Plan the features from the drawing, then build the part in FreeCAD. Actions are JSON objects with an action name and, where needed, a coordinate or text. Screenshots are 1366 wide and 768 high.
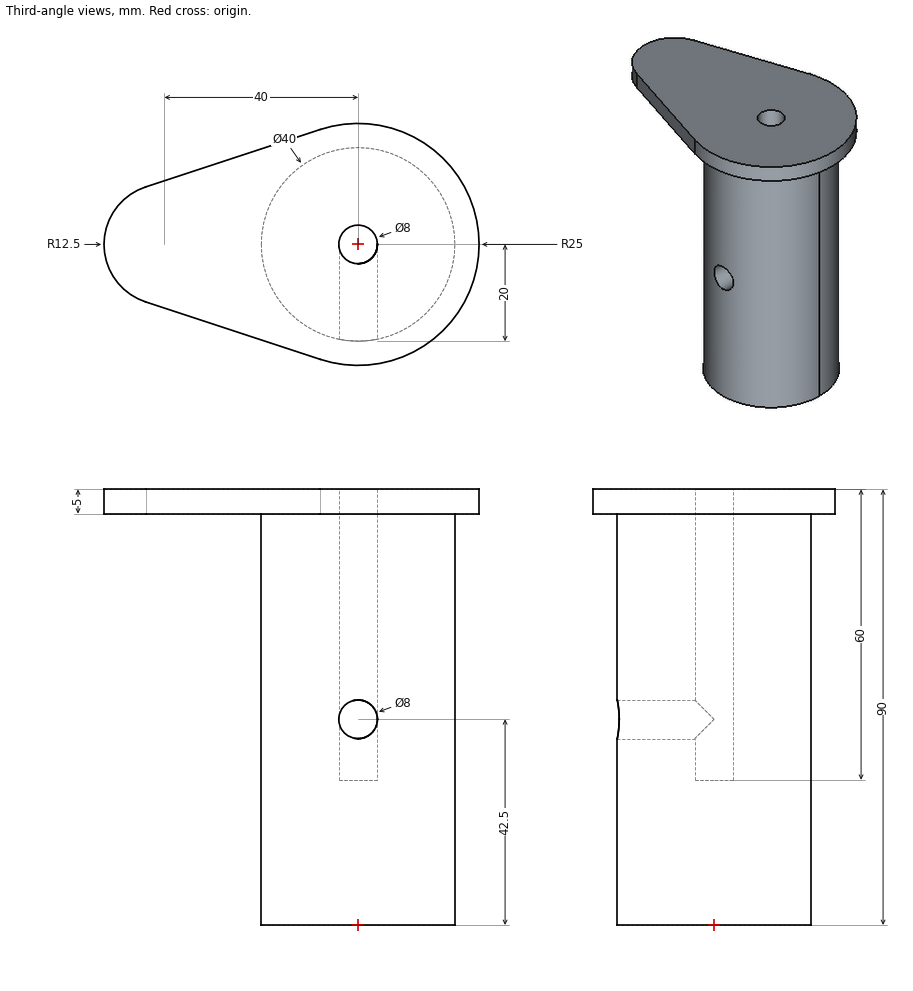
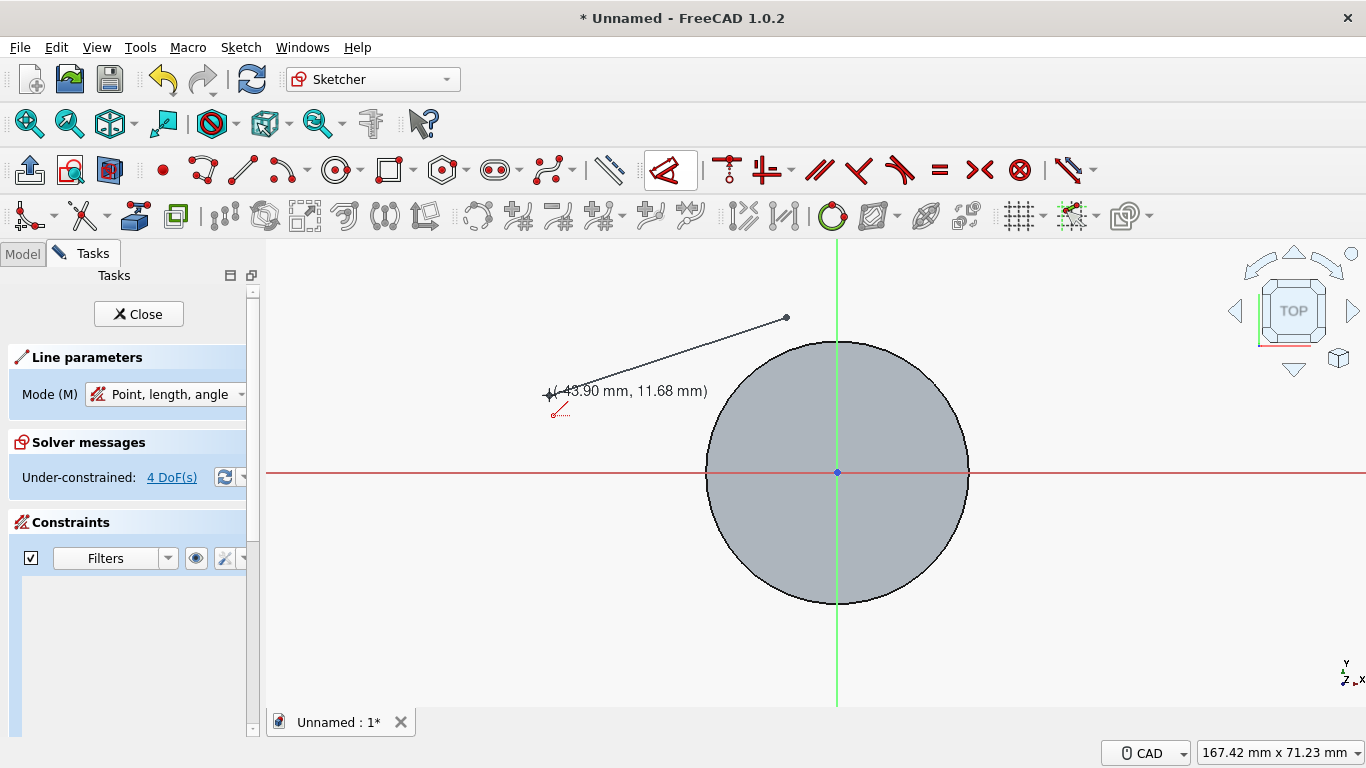
{"action": "left_click", "coordinate": [549, 551]}
{"action": "left_click", "coordinate": [786, 629]}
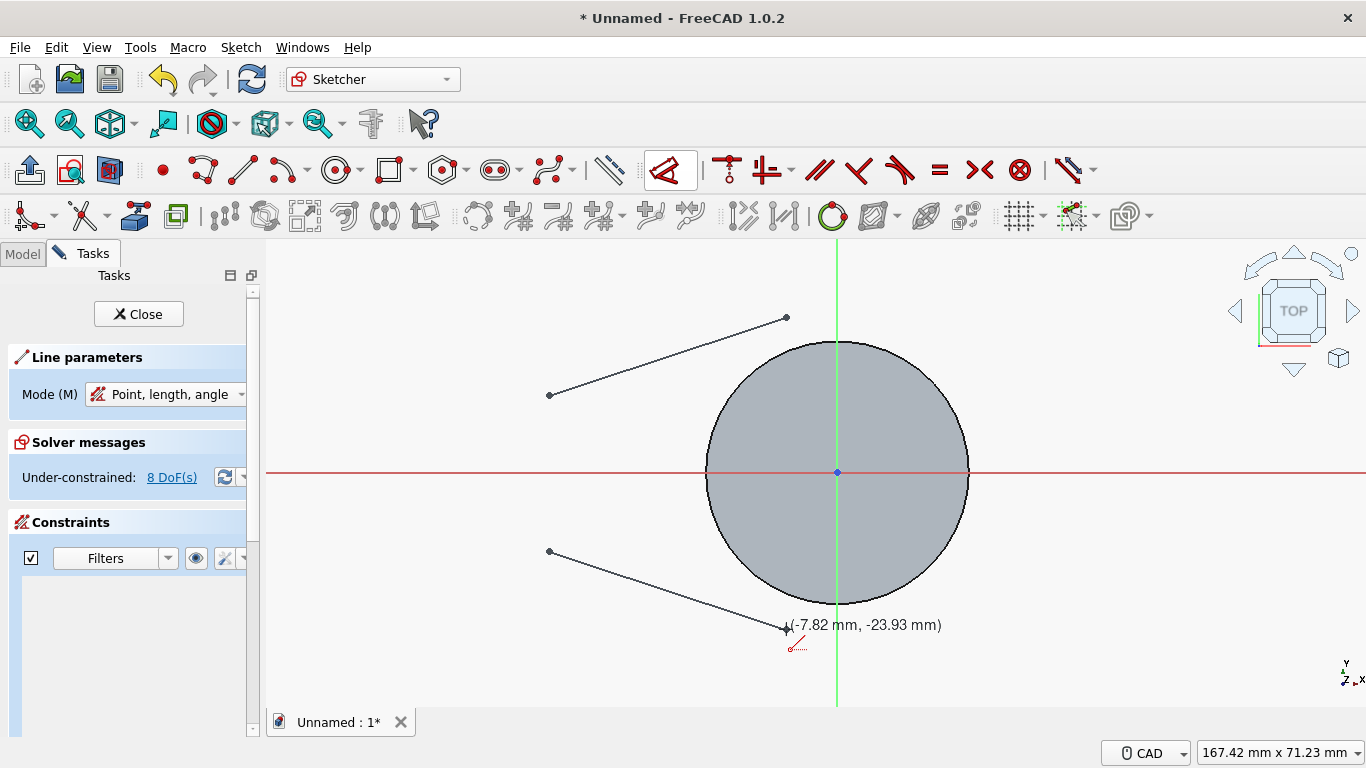
{"action": "key", "text": "g 3 a"}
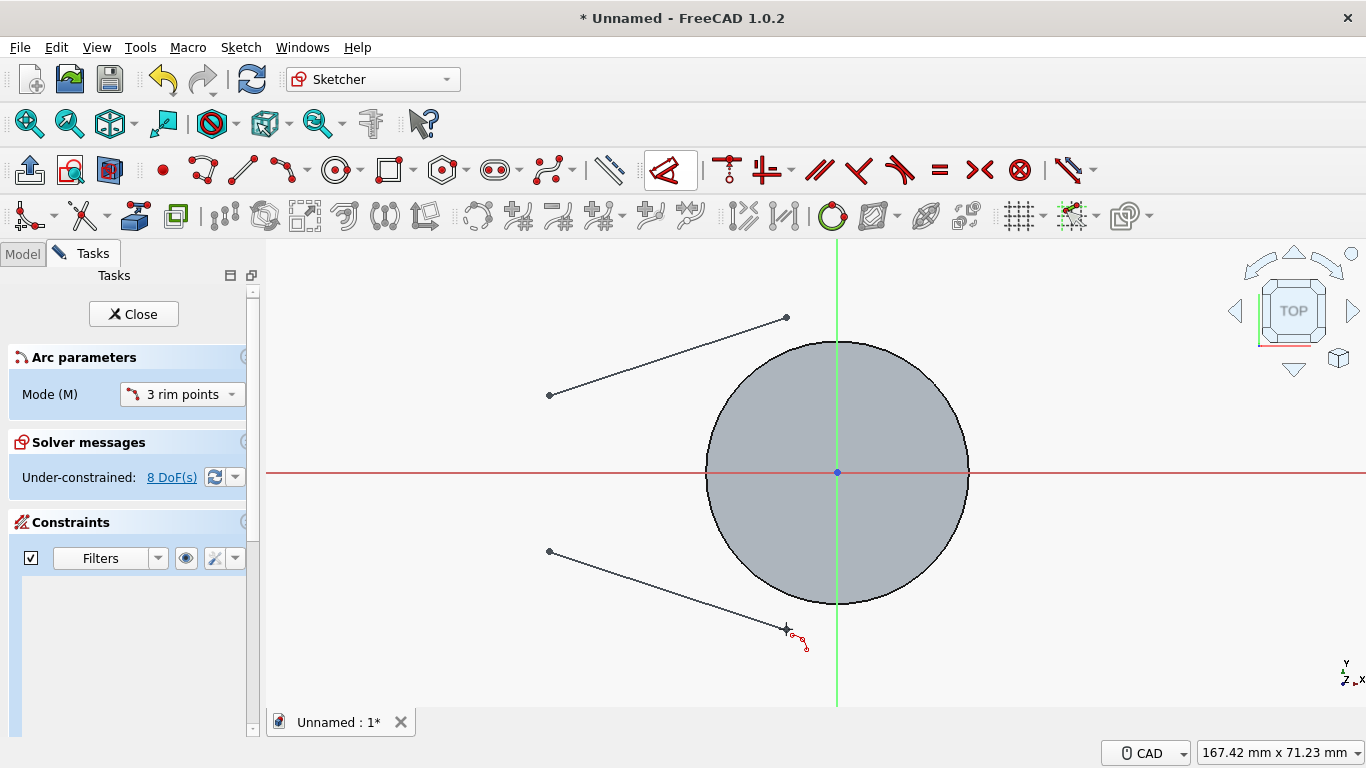
{"action": "left_click", "coordinate": [549, 396]}
{"action": "left_click", "coordinate": [549, 552]}
{"action": "left_click", "coordinate": [495, 452]}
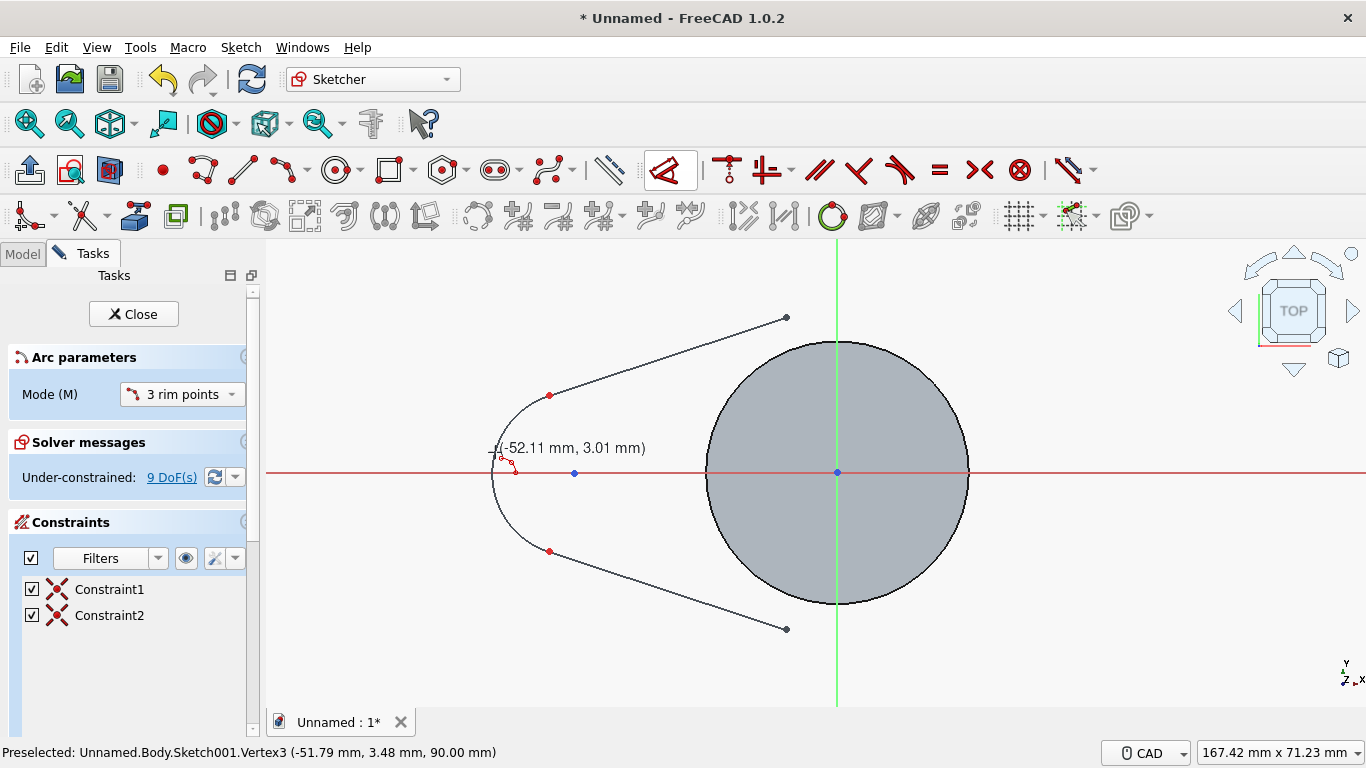
{"action": "left_click", "coordinate": [786, 630]}
{"action": "left_click", "coordinate": [786, 318]}
{"action": "left_click", "coordinate": [990, 533]}
{"action": "key", "text": "Escape"}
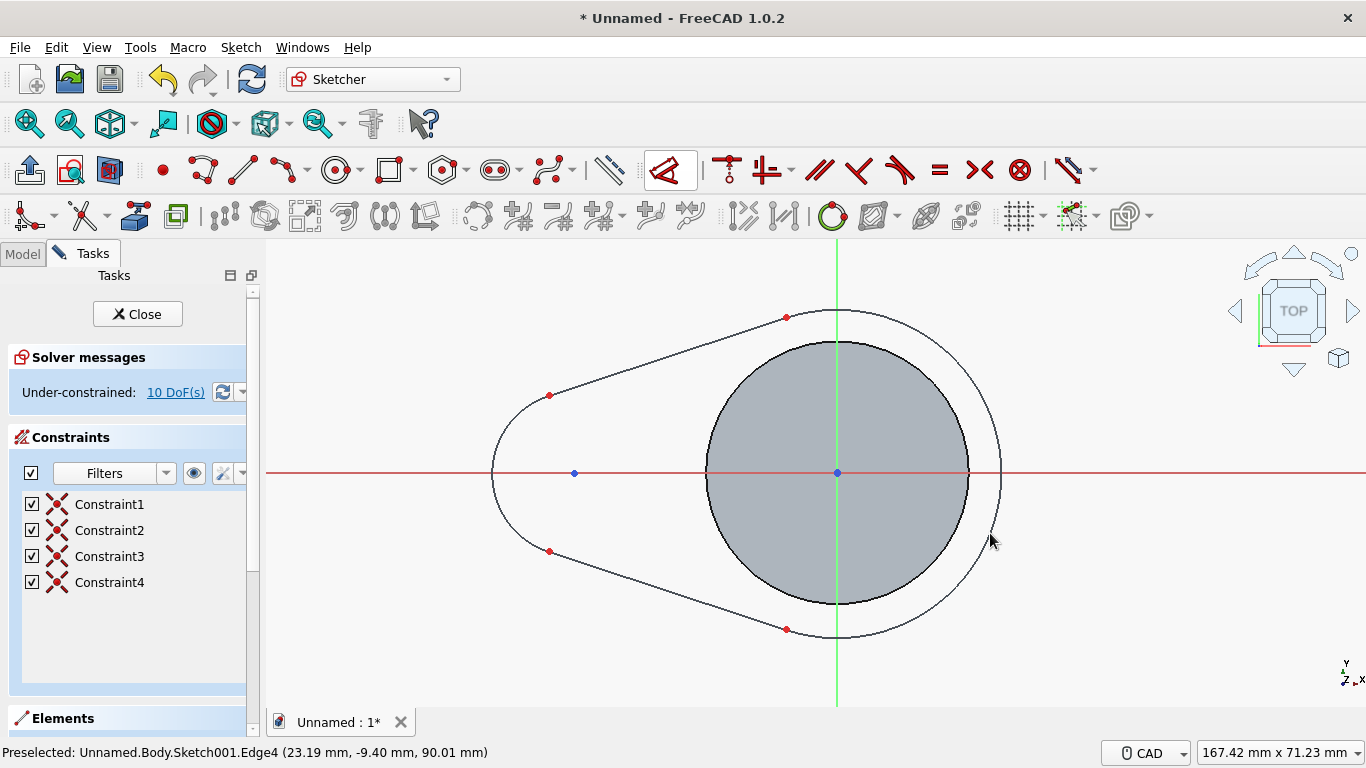
{"action": "left_click", "coordinate": [715, 341]}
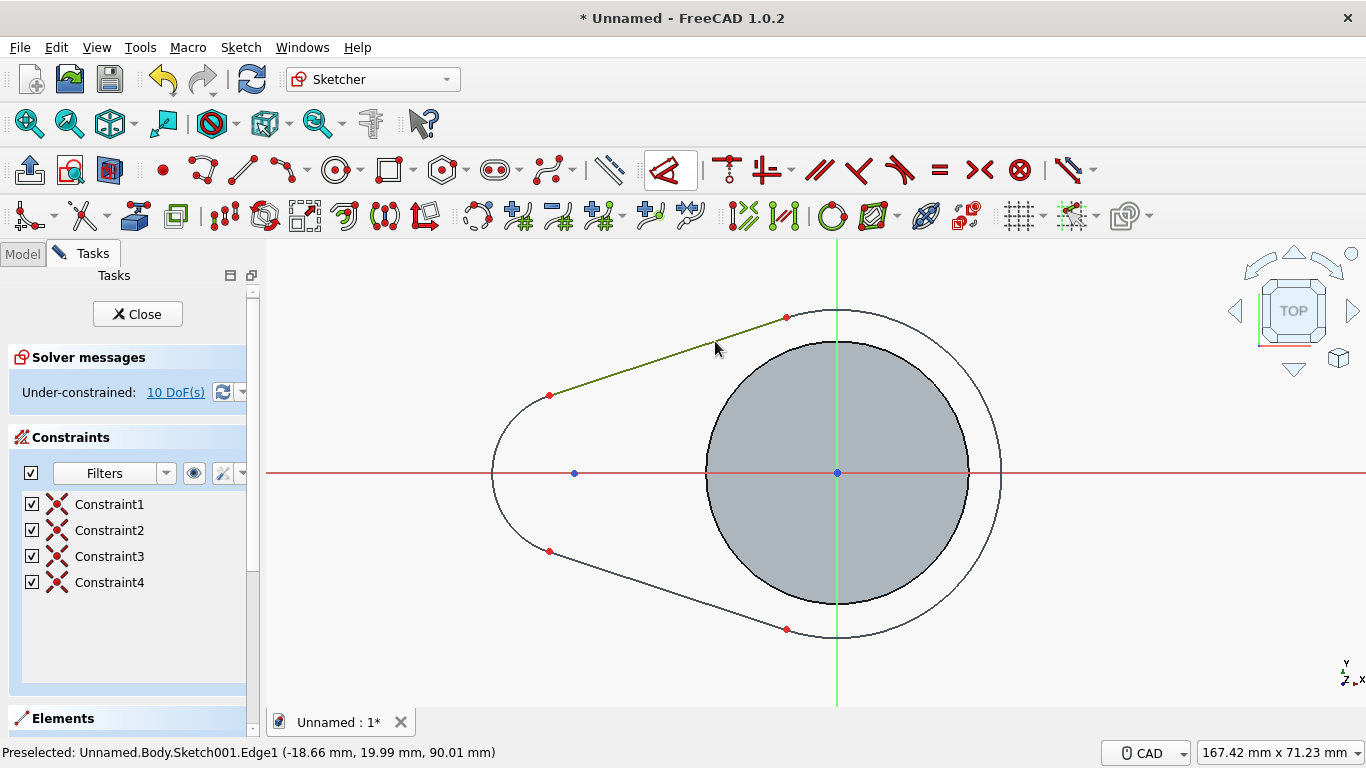
{"action": "left_click", "coordinate": [502, 434]}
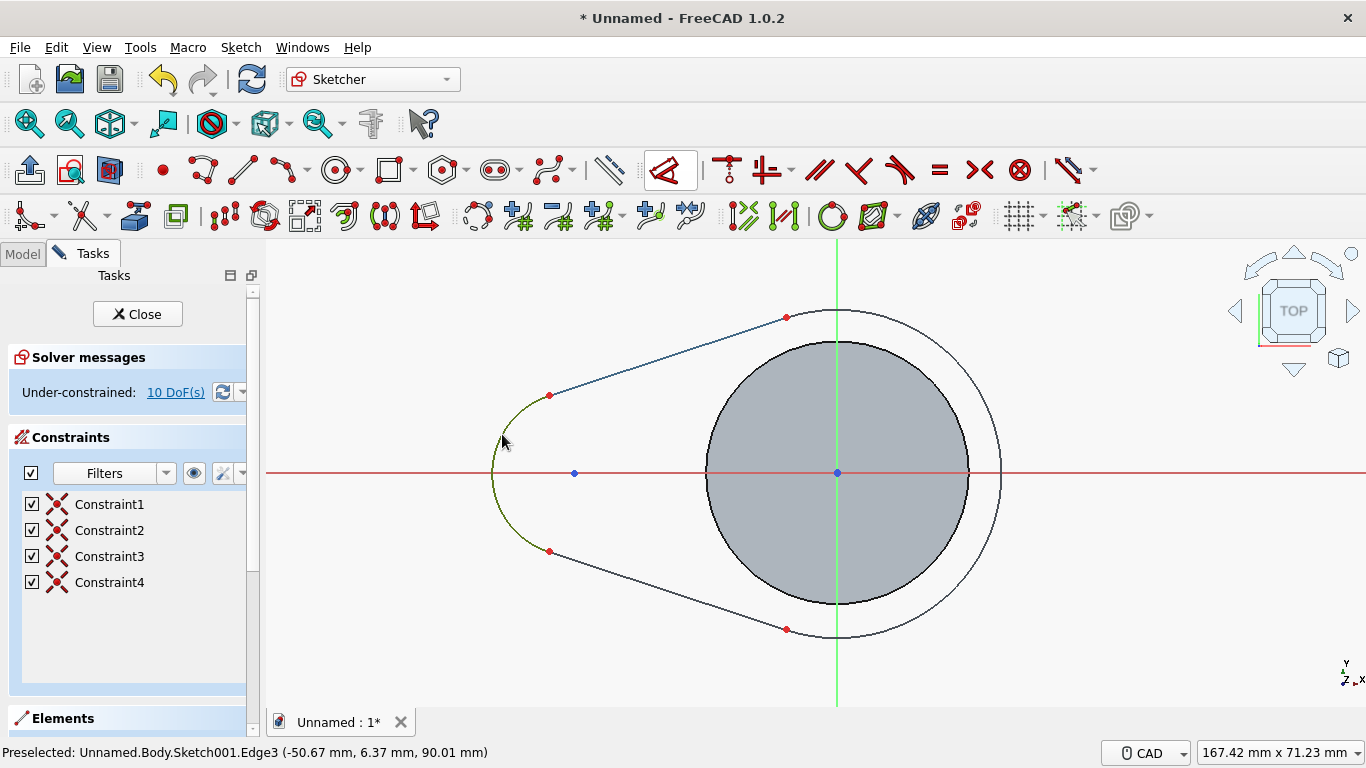
{"action": "key", "text": "t"}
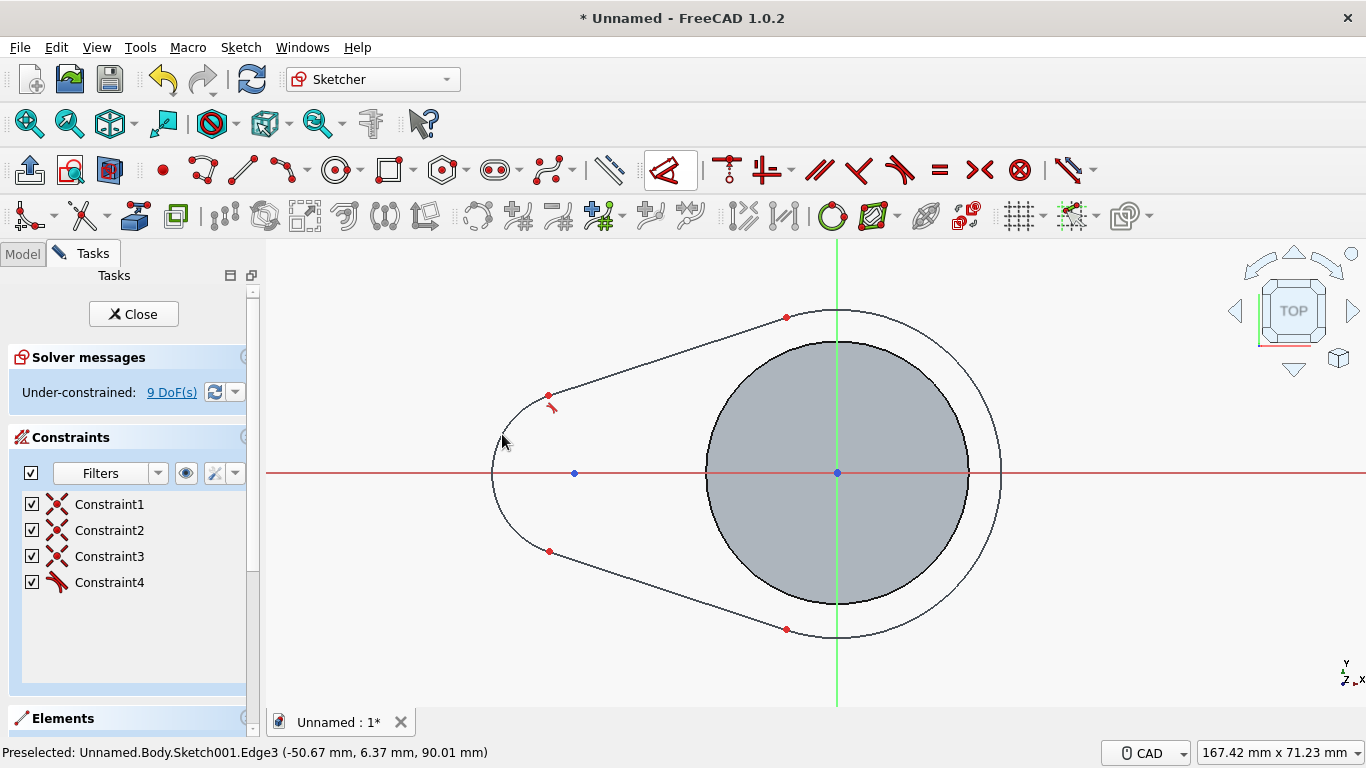
{"action": "left_click", "coordinate": [715, 341]}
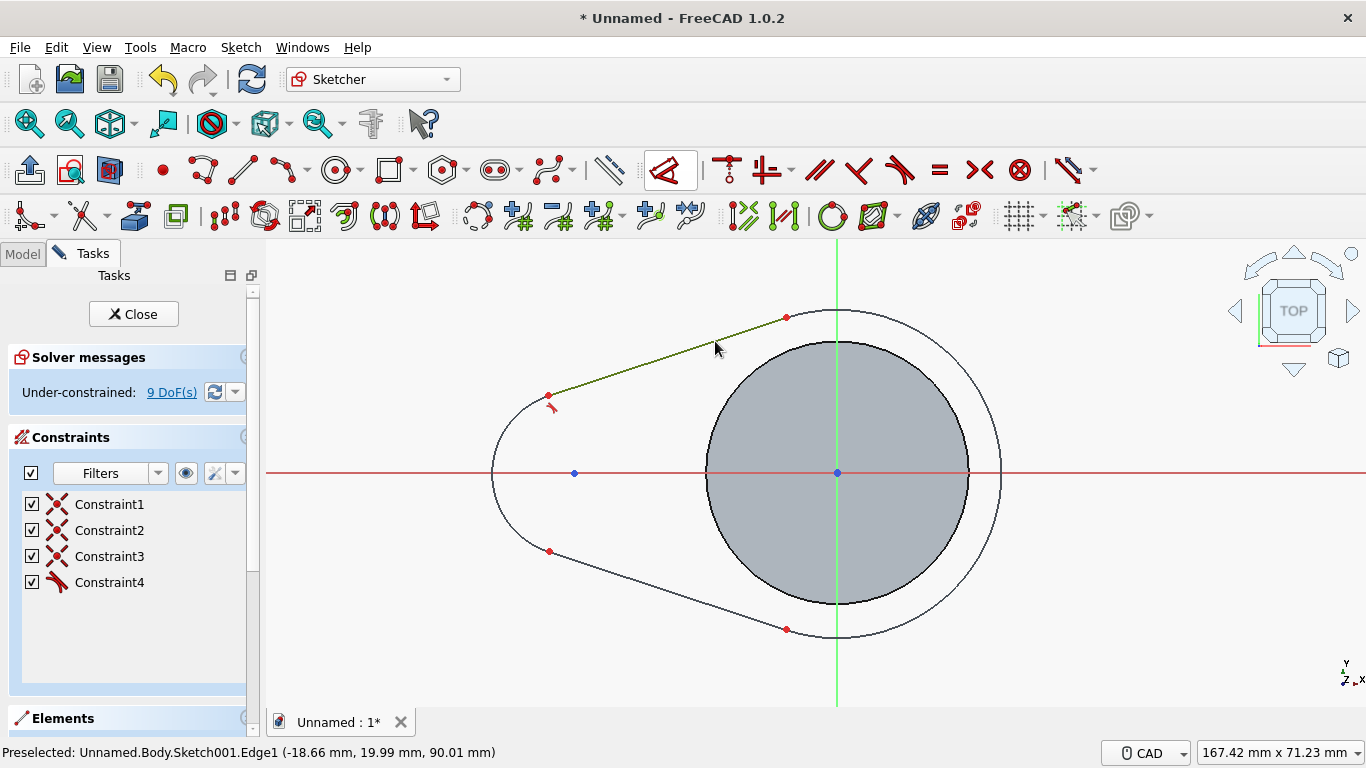
{"action": "left_click", "coordinate": [957, 587]}